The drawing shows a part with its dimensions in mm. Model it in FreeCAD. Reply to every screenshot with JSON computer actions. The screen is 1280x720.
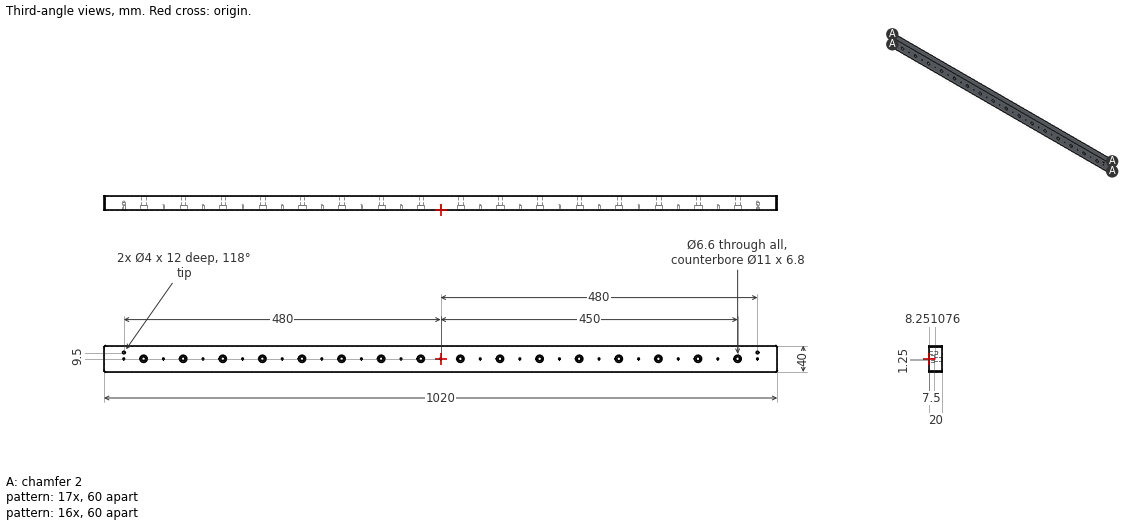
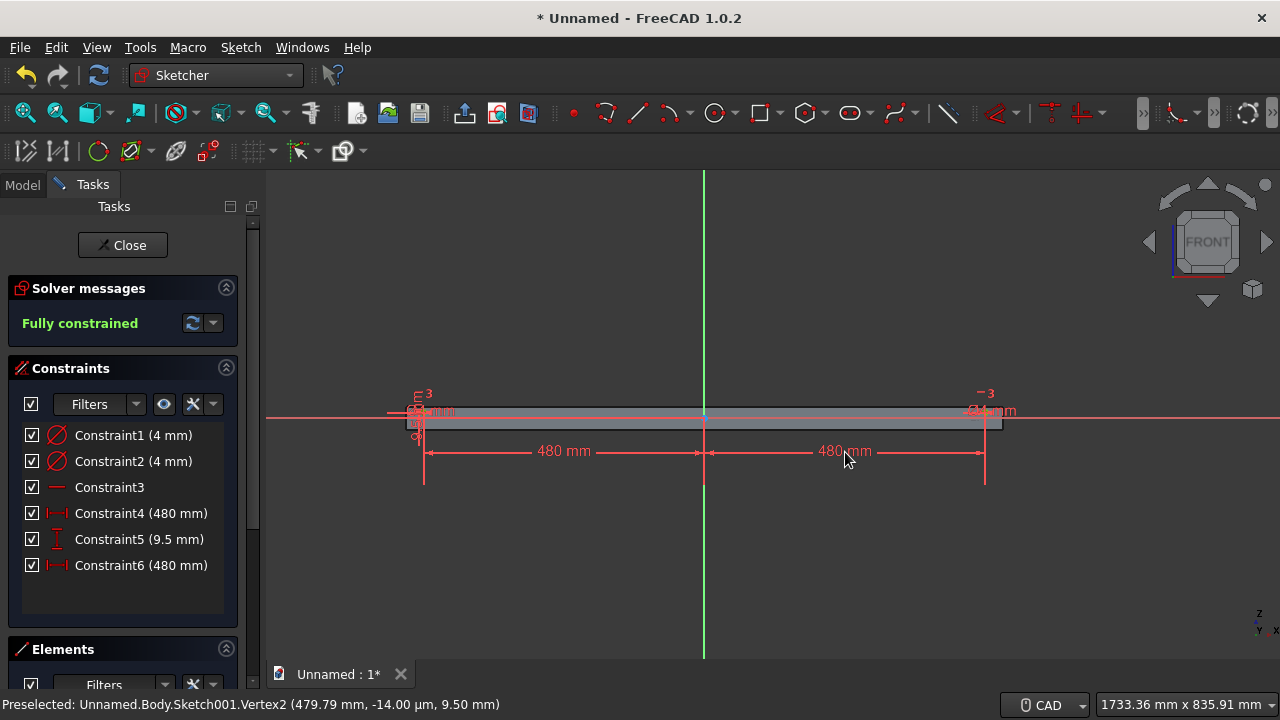
{"action": "left_click", "coordinate": [123, 245]}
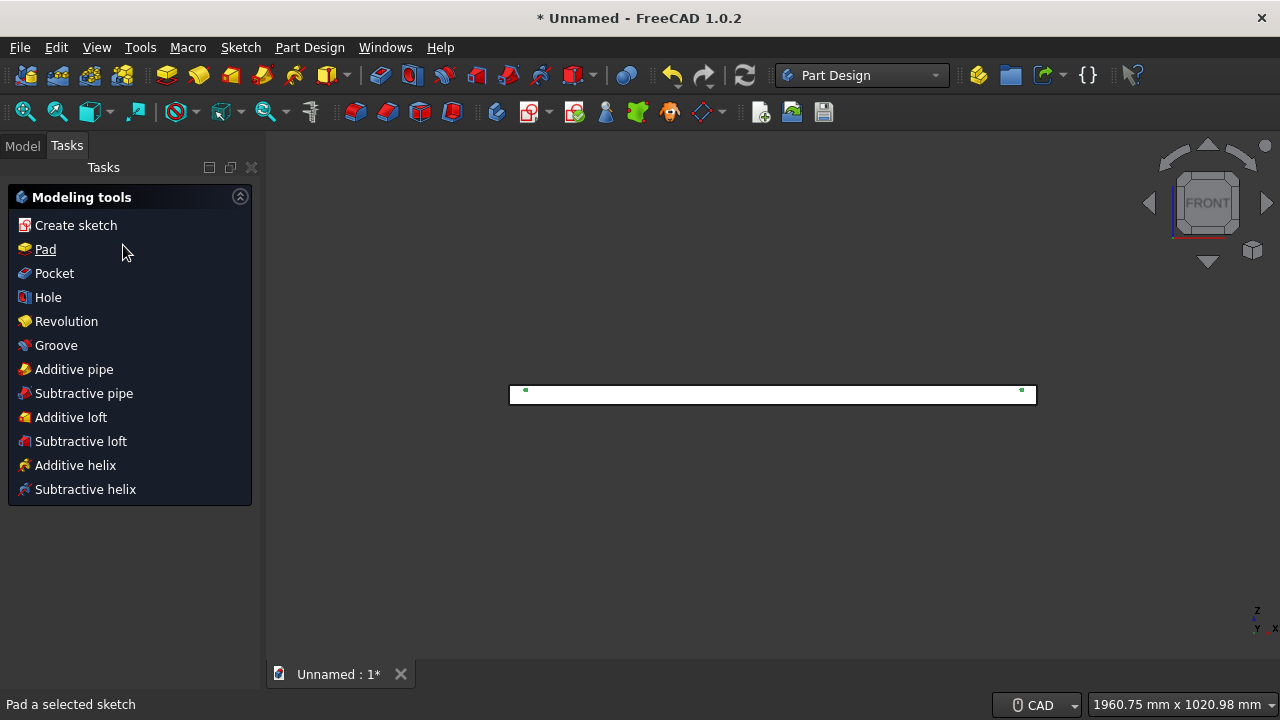
{"action": "left_click", "coordinate": [414, 76]}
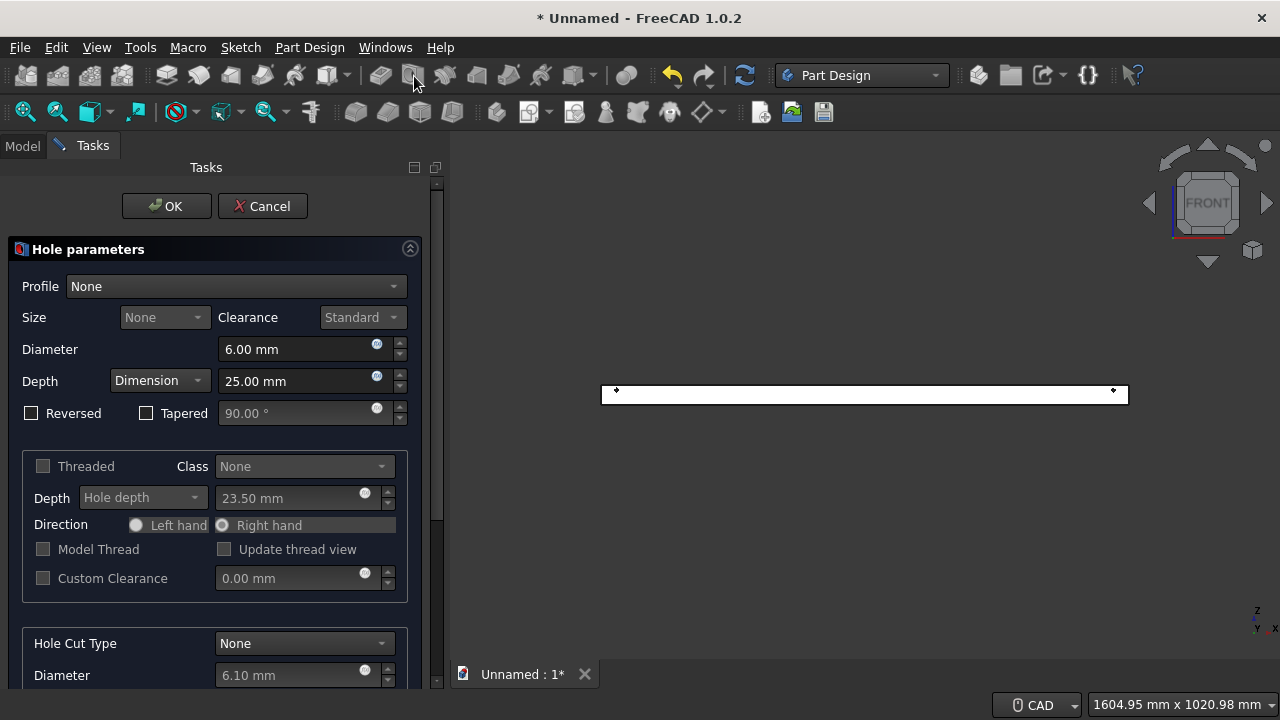
{"action": "triple_click", "coordinate": [305, 349]}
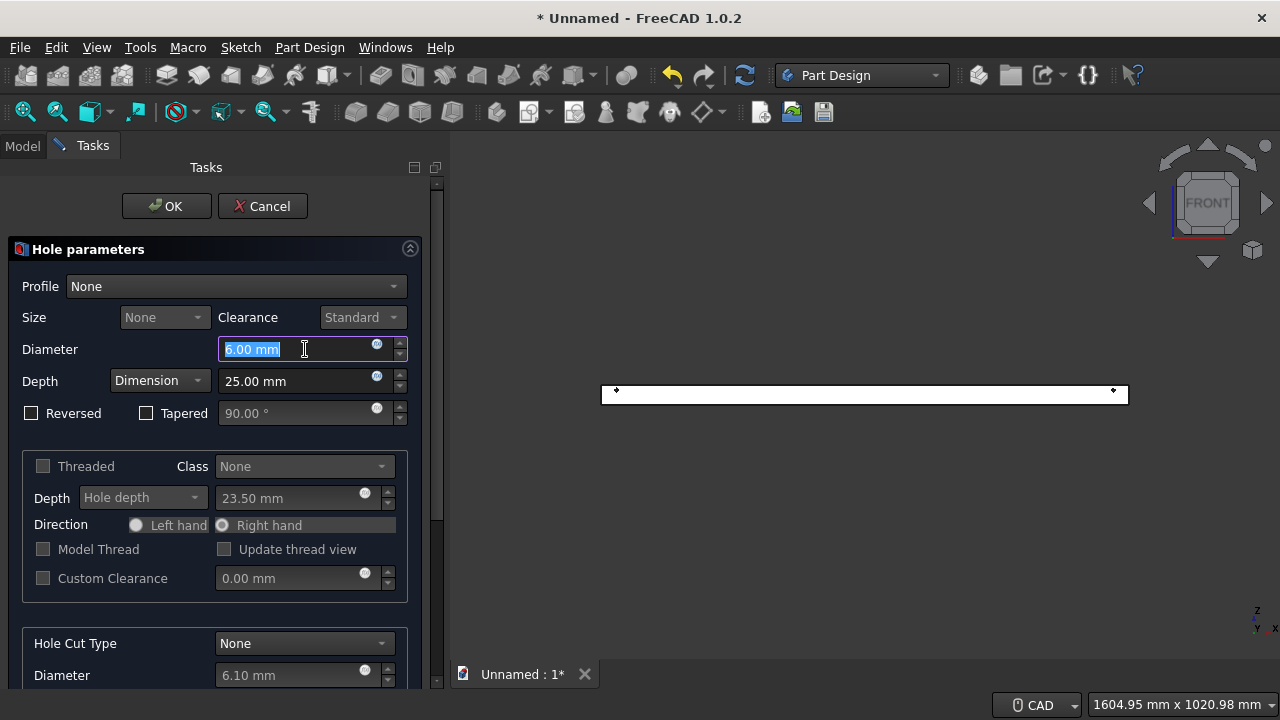
{"action": "type", "text": "4"}
{"action": "key", "text": "Tab"}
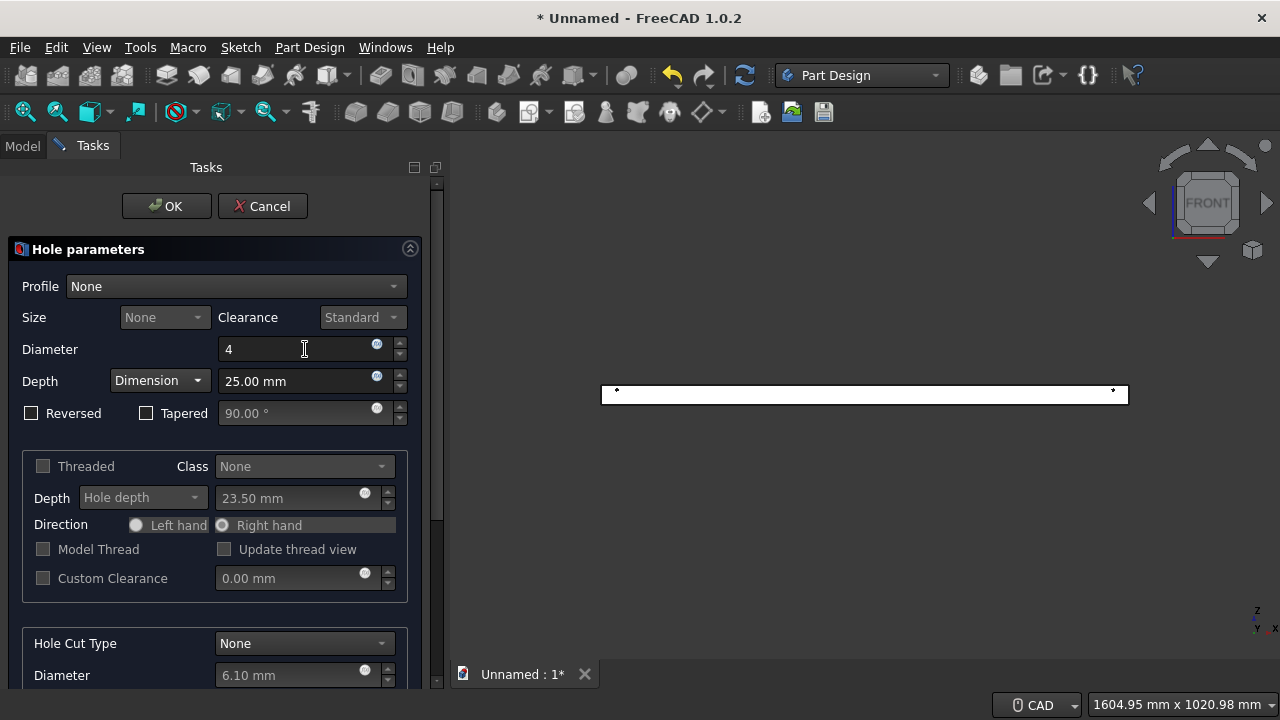
{"action": "triple_click", "coordinate": [305, 381]}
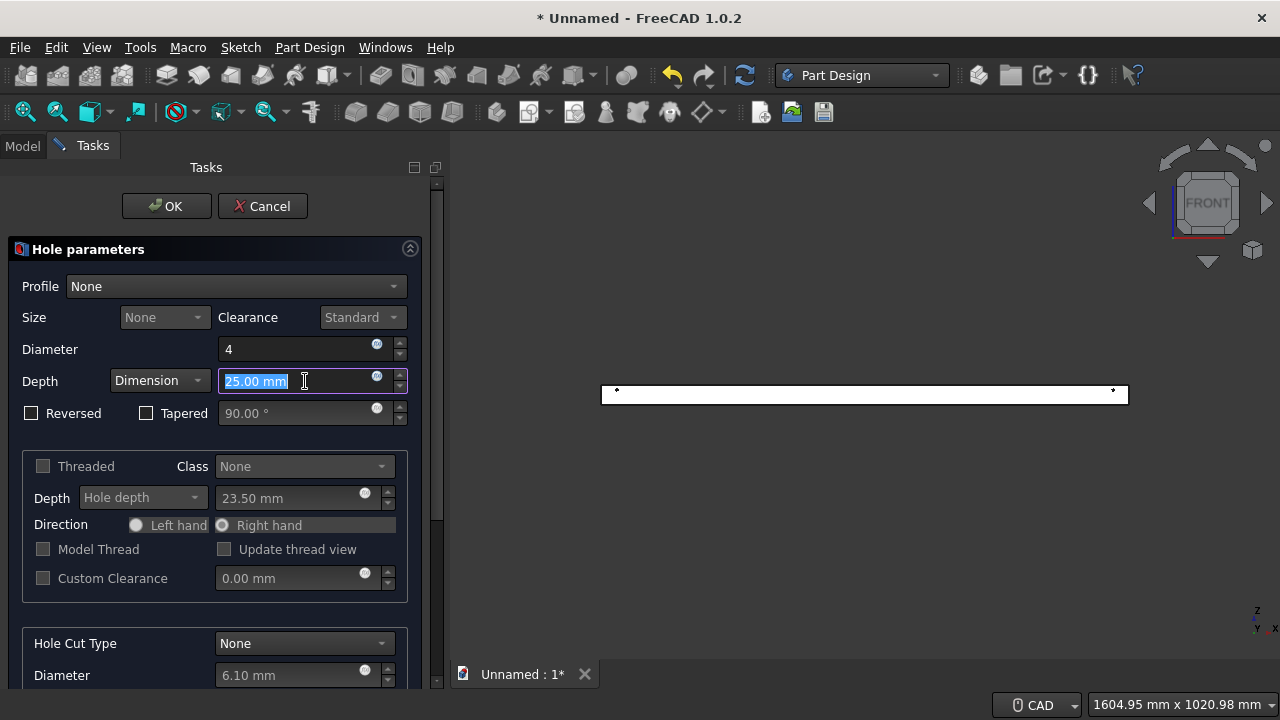
{"action": "type", "text": "12"}
{"action": "key", "text": "Tab"}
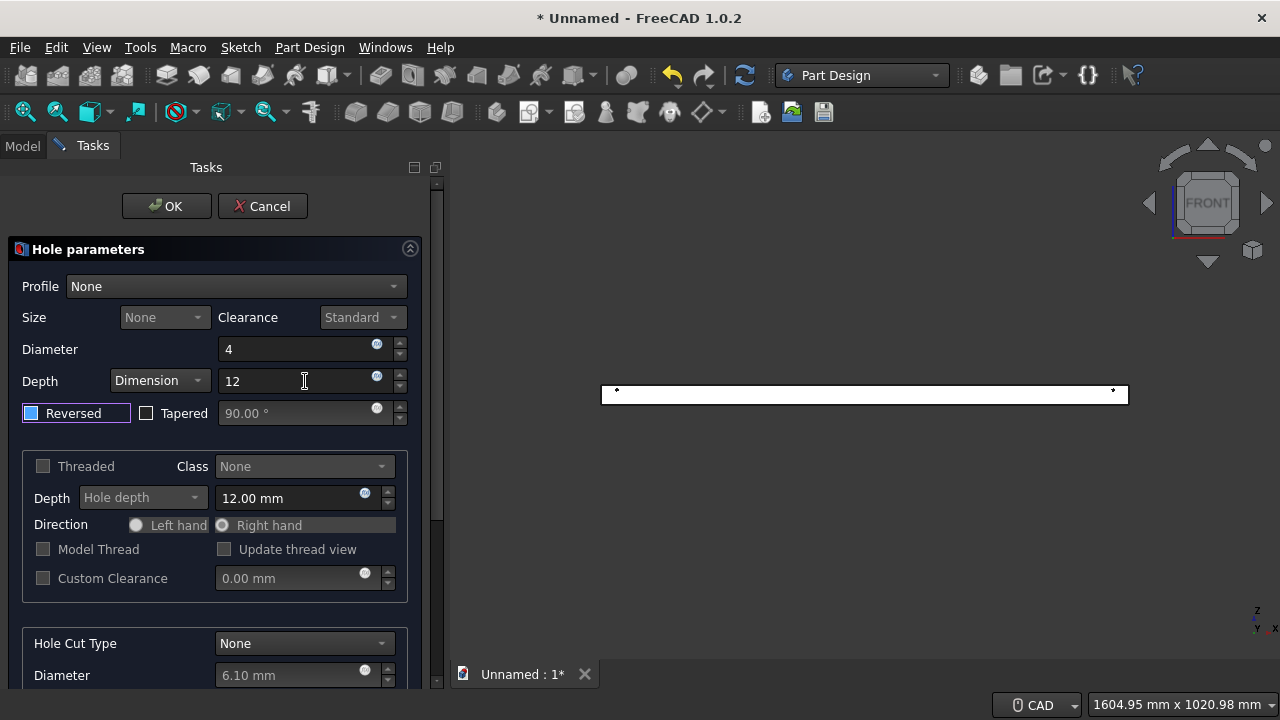
{"action": "left_click", "coordinate": [167, 206]}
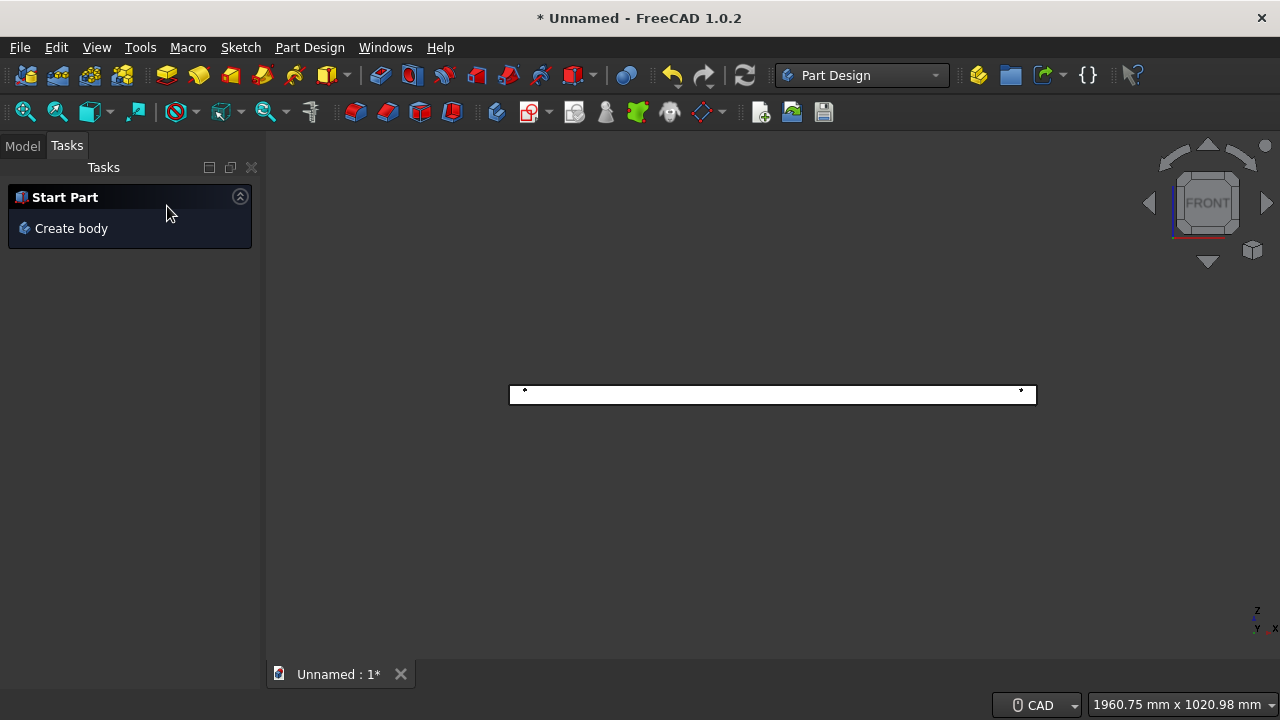
{"action": "left_click", "coordinate": [23, 145]}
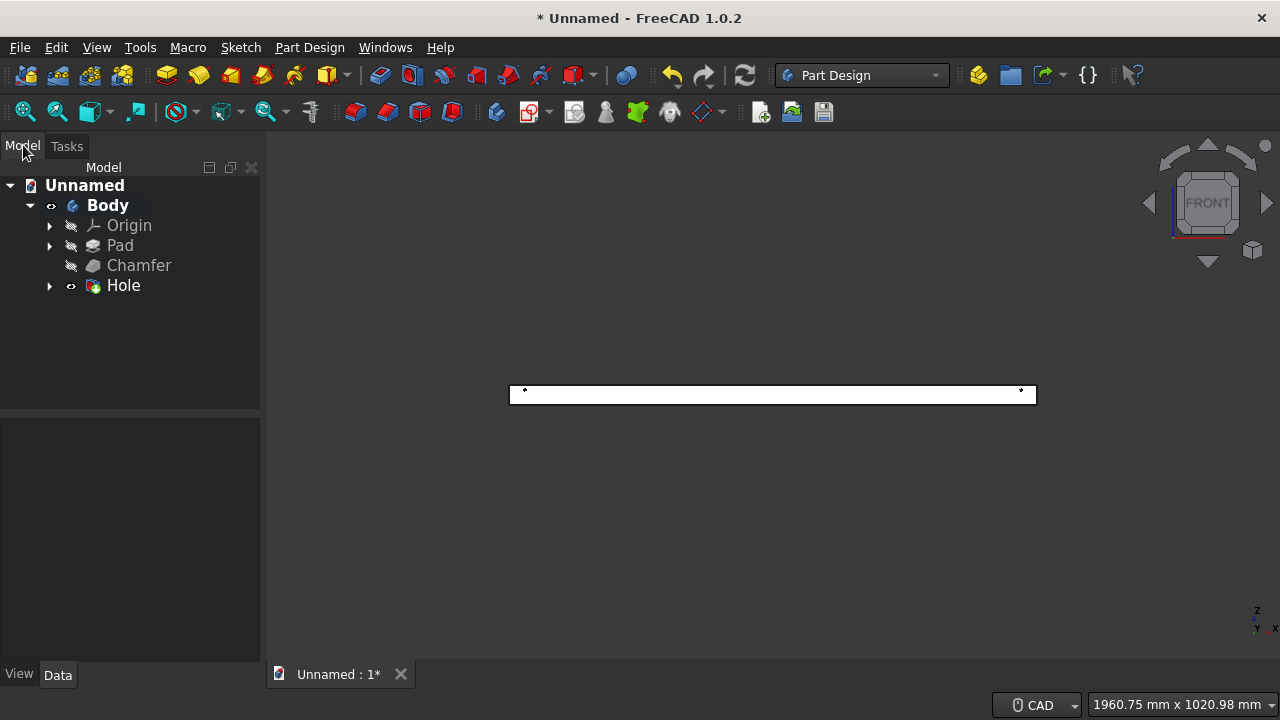
{"action": "left_click", "coordinate": [50, 226]}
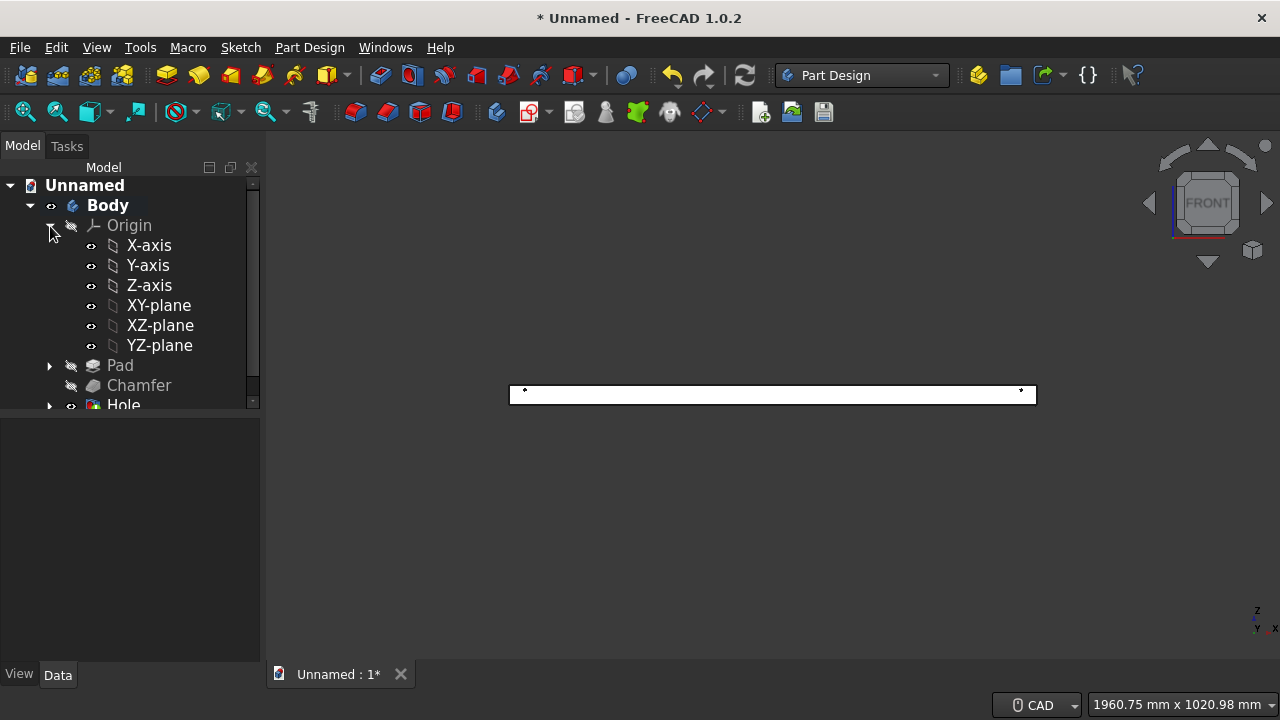
{"action": "left_click", "coordinate": [136, 346]}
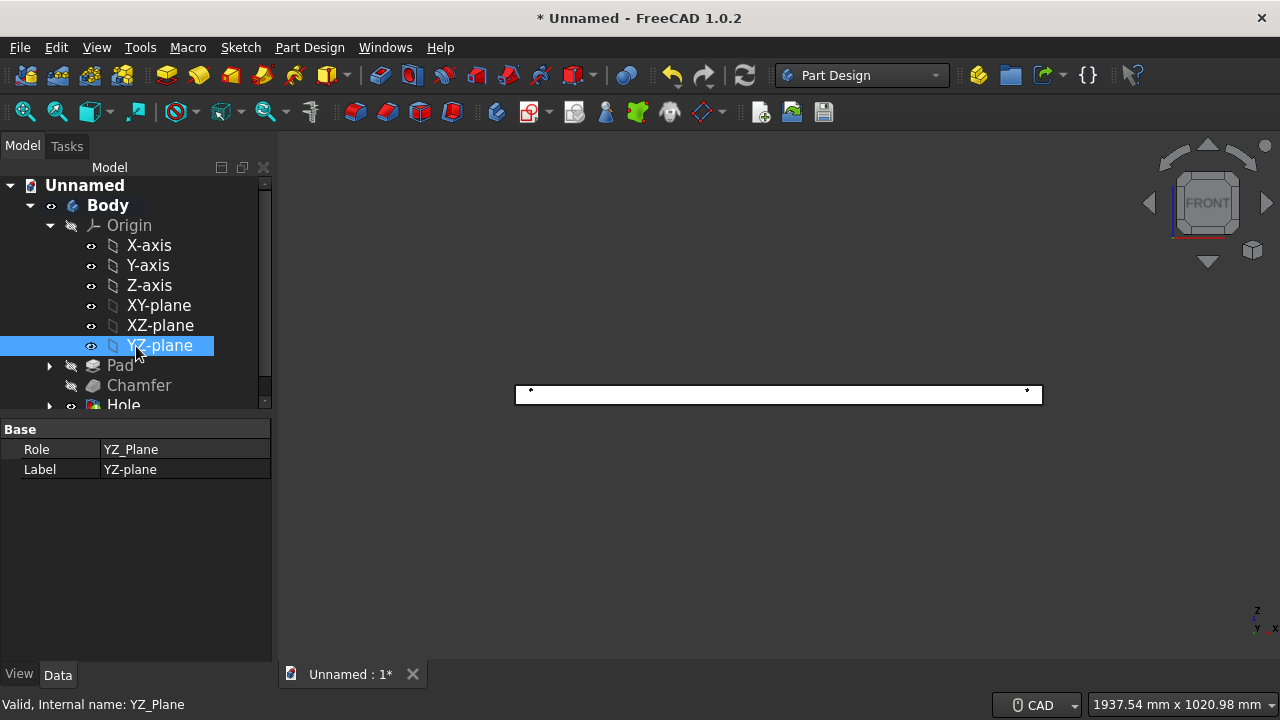
{"action": "left_click", "coordinate": [702, 112]}